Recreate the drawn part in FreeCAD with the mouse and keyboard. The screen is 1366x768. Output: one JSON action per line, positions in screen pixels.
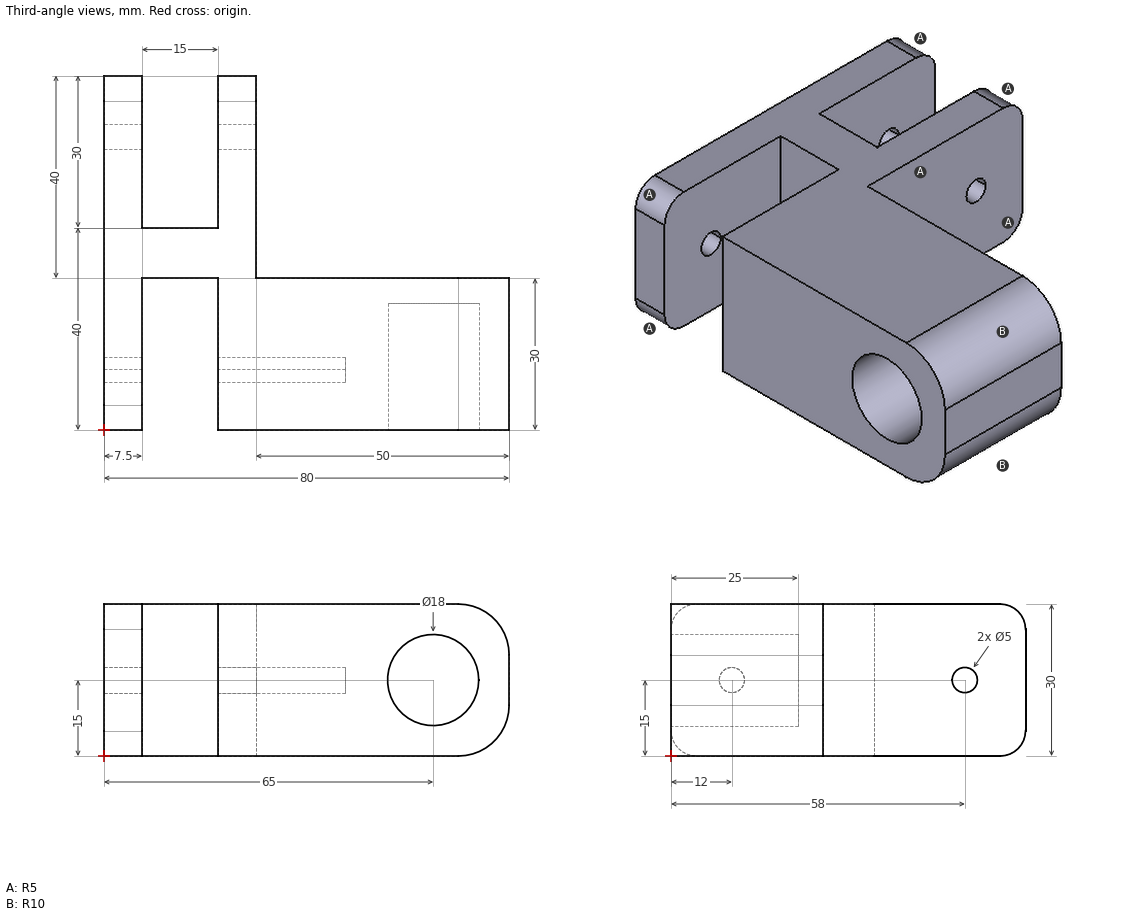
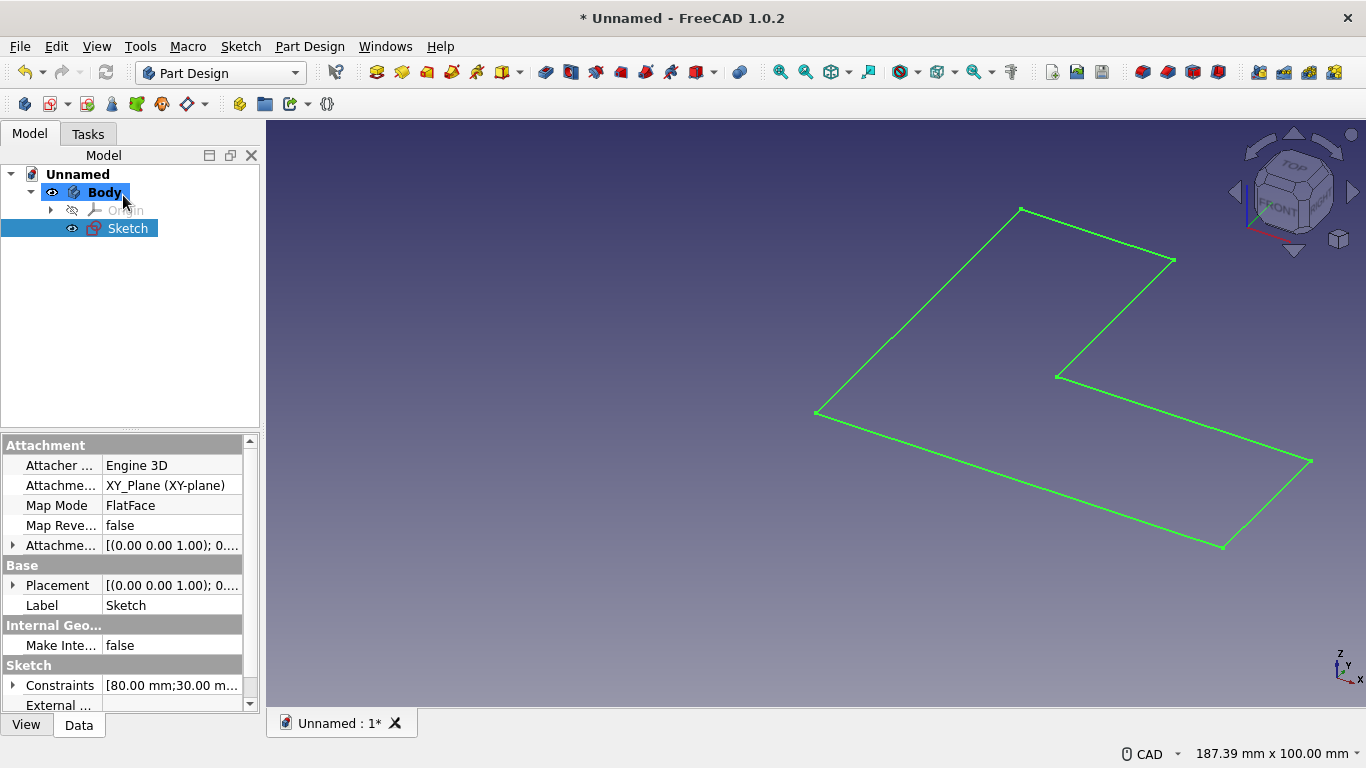
{"action": "left_click", "coordinate": [377, 72]}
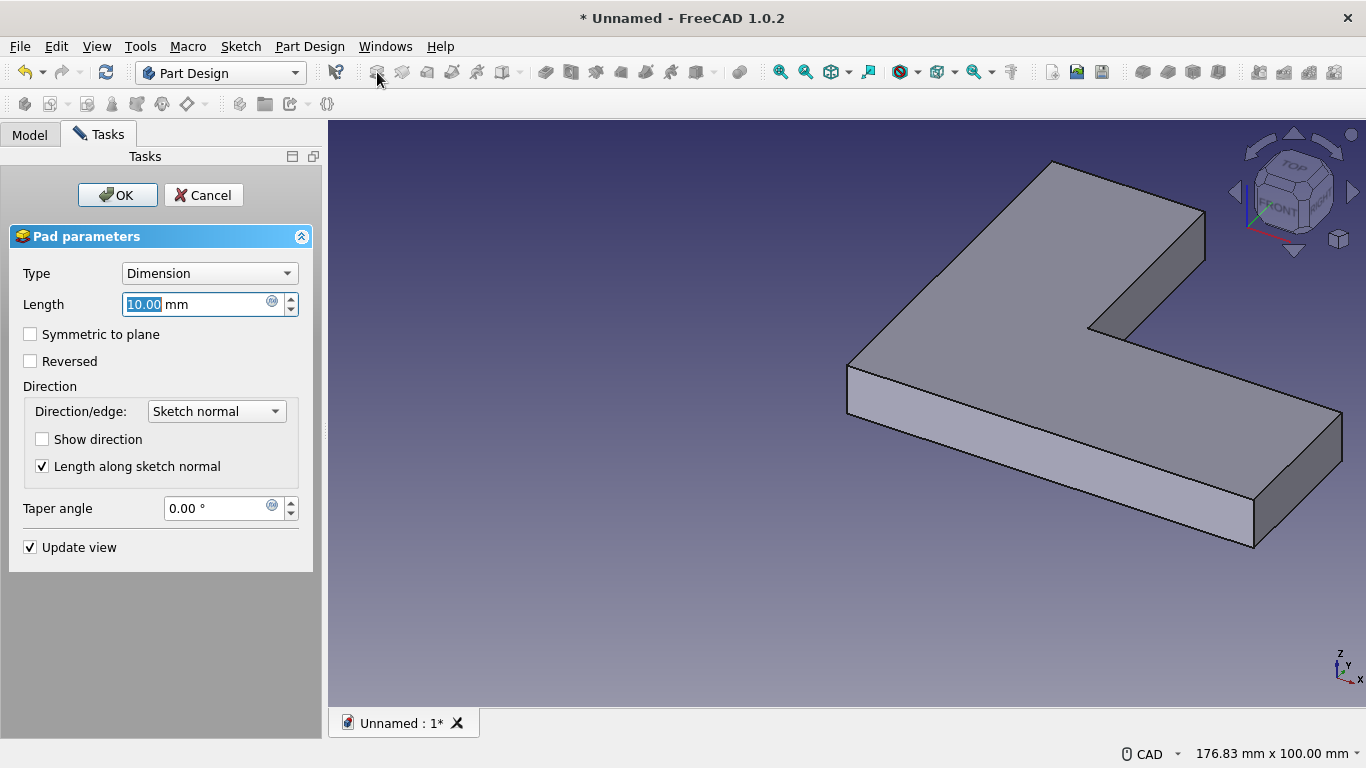
{"action": "type", "text": "30"}
{"action": "key", "text": "Tab"}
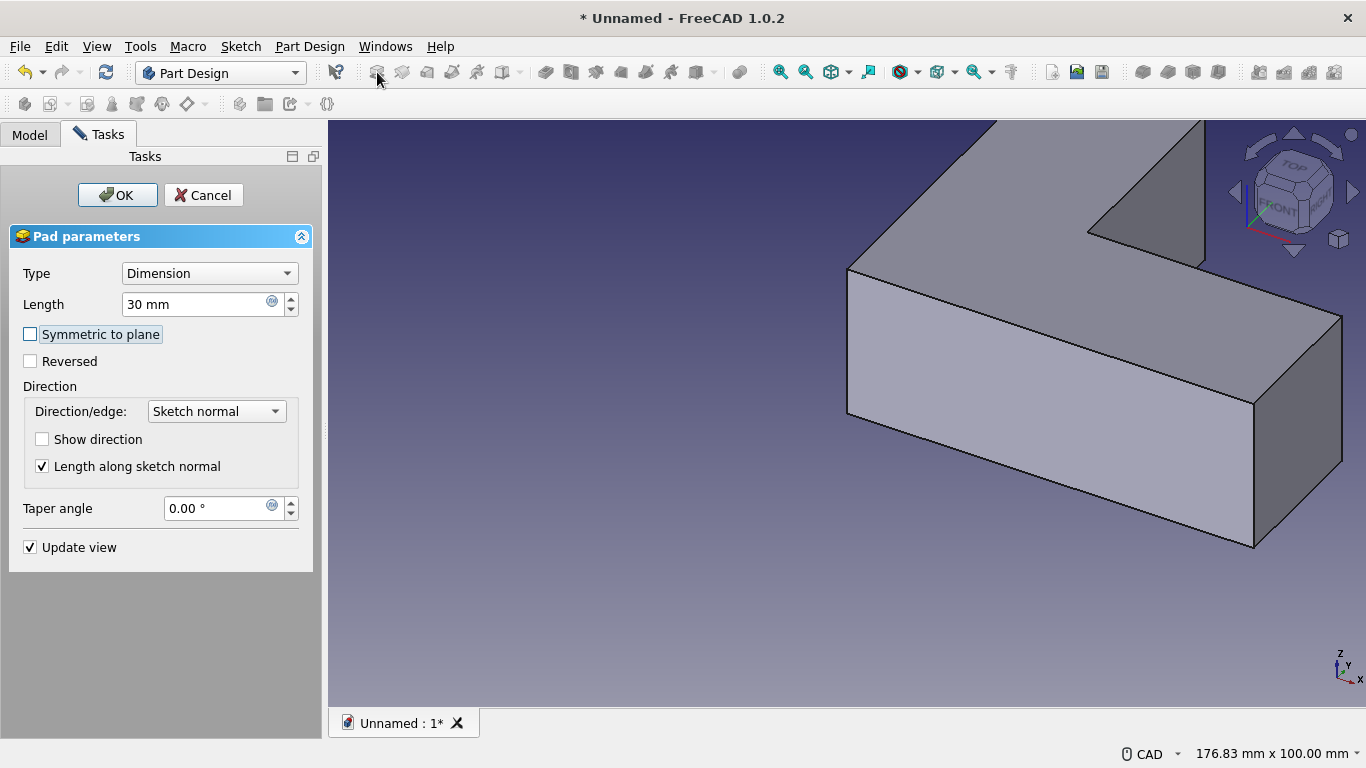
{"action": "left_click", "coordinate": [118, 195]}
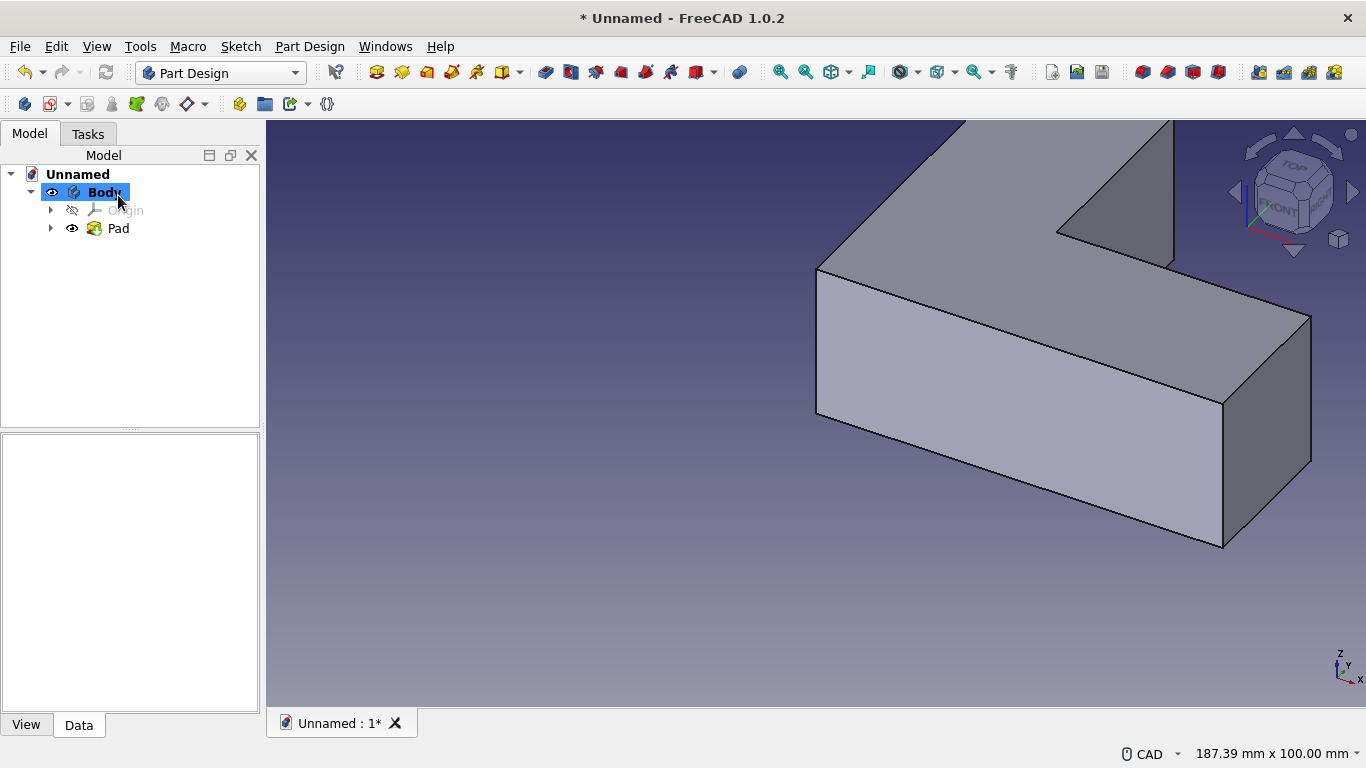
{"action": "left_click", "coordinate": [781, 72]}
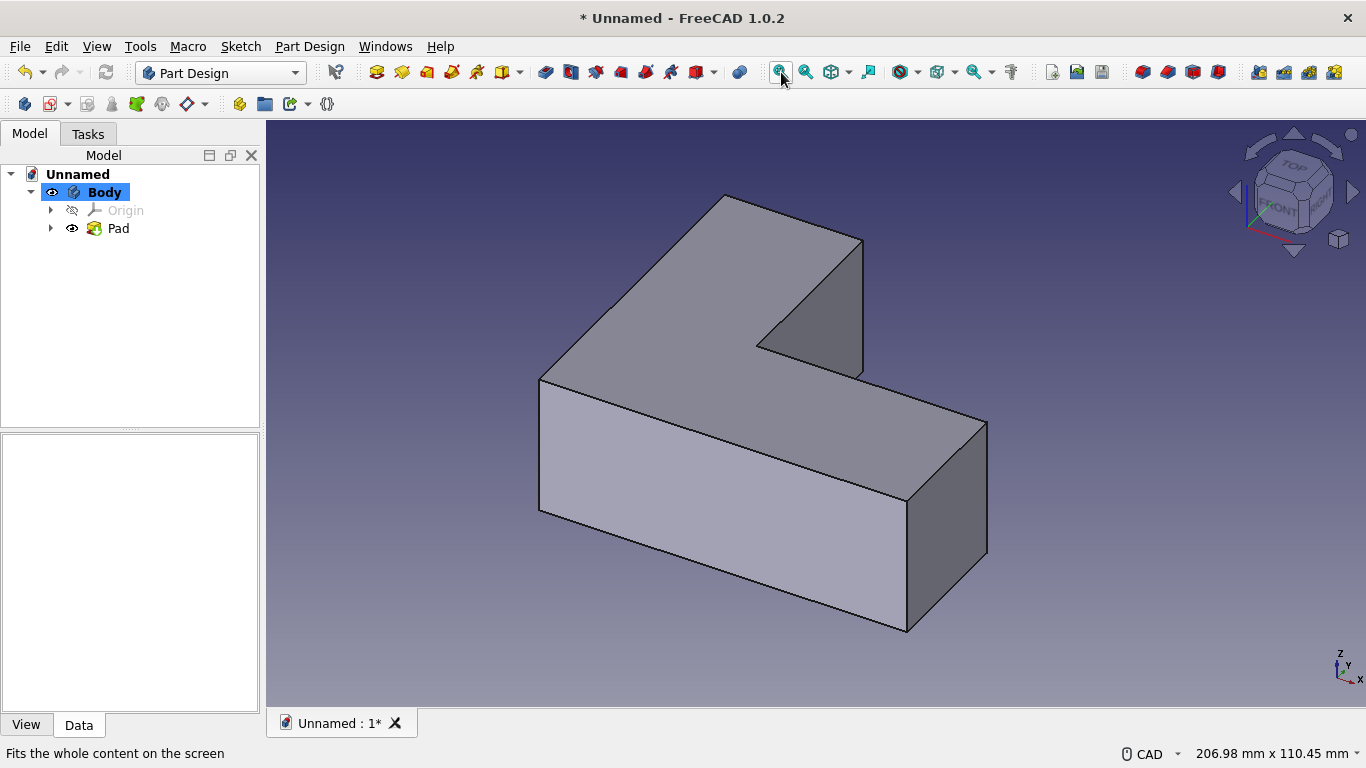
{"action": "left_click", "coordinate": [828, 540]}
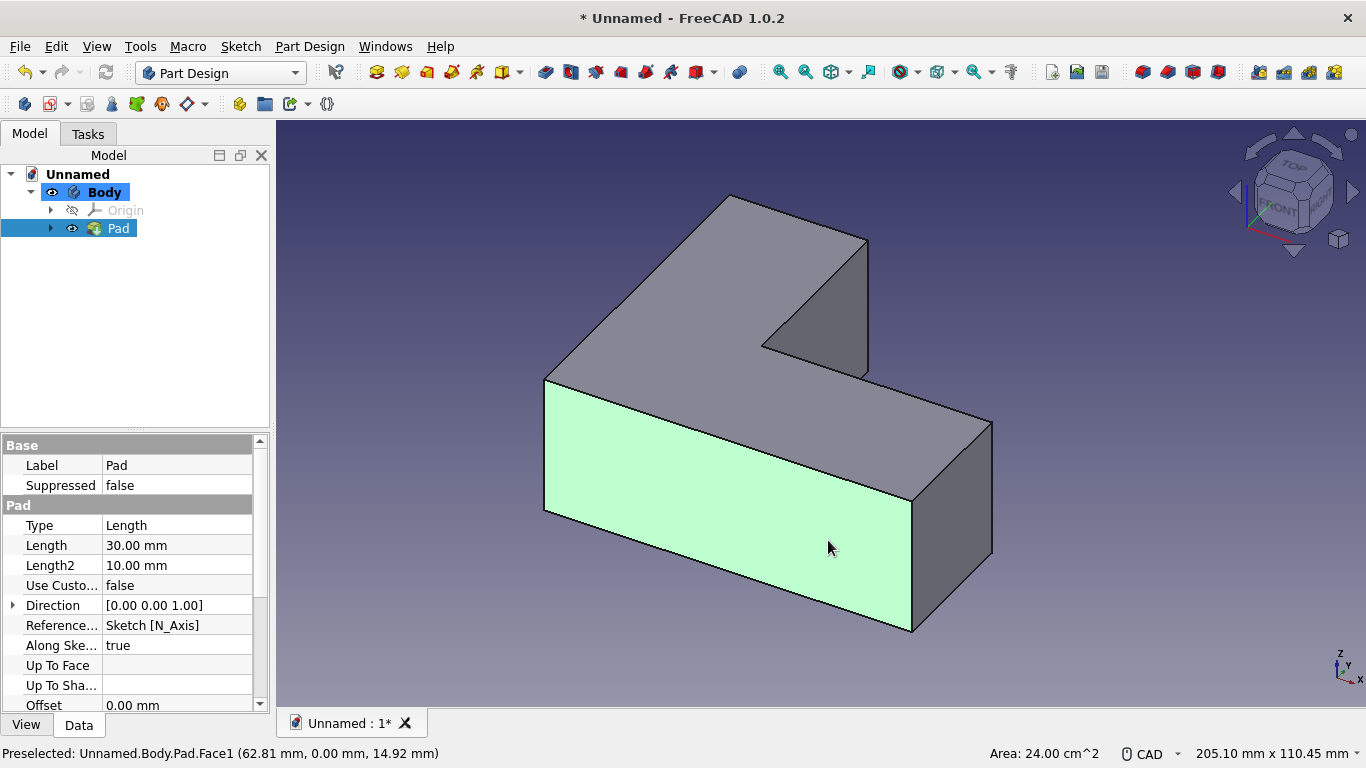
{"action": "left_click", "coordinate": [50, 104]}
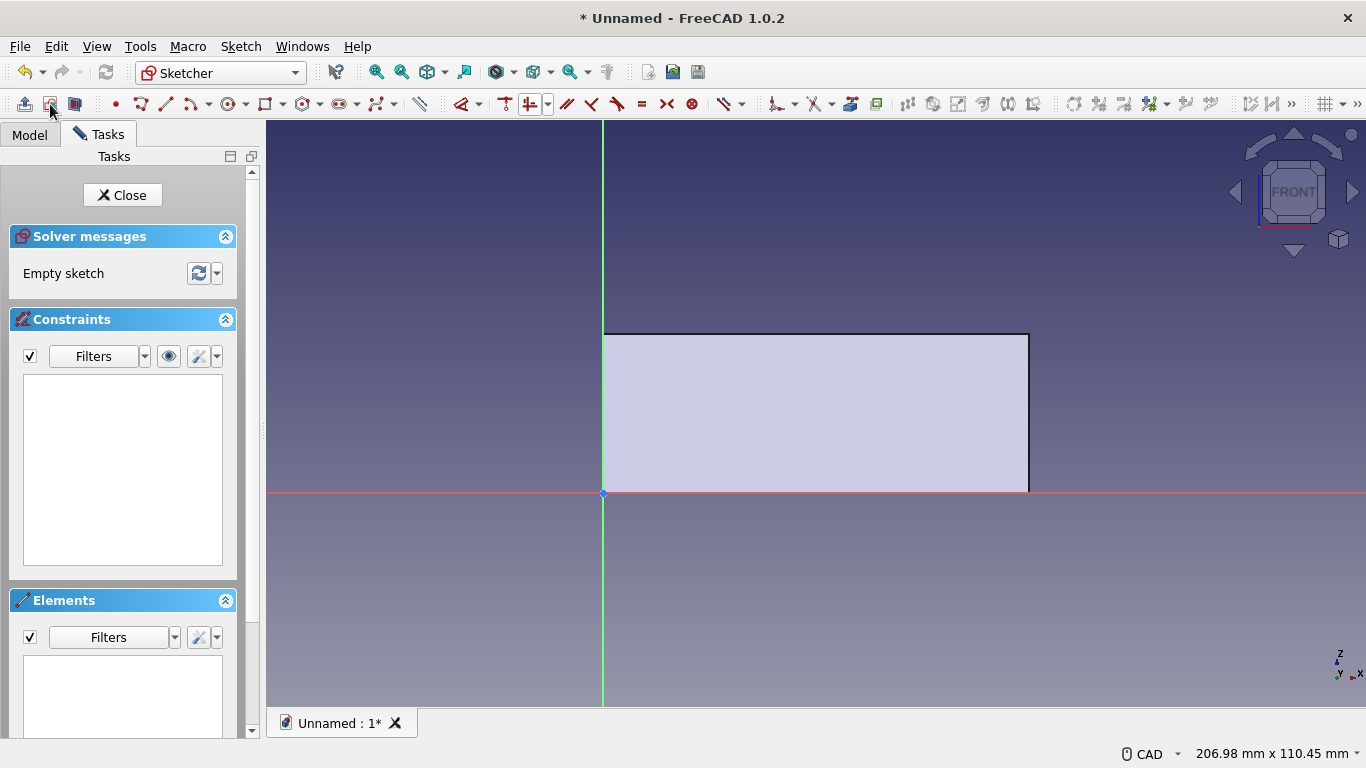
{"action": "scroll", "coordinate": [1015, 414], "scroll_direction": "up", "scroll_amount": 7}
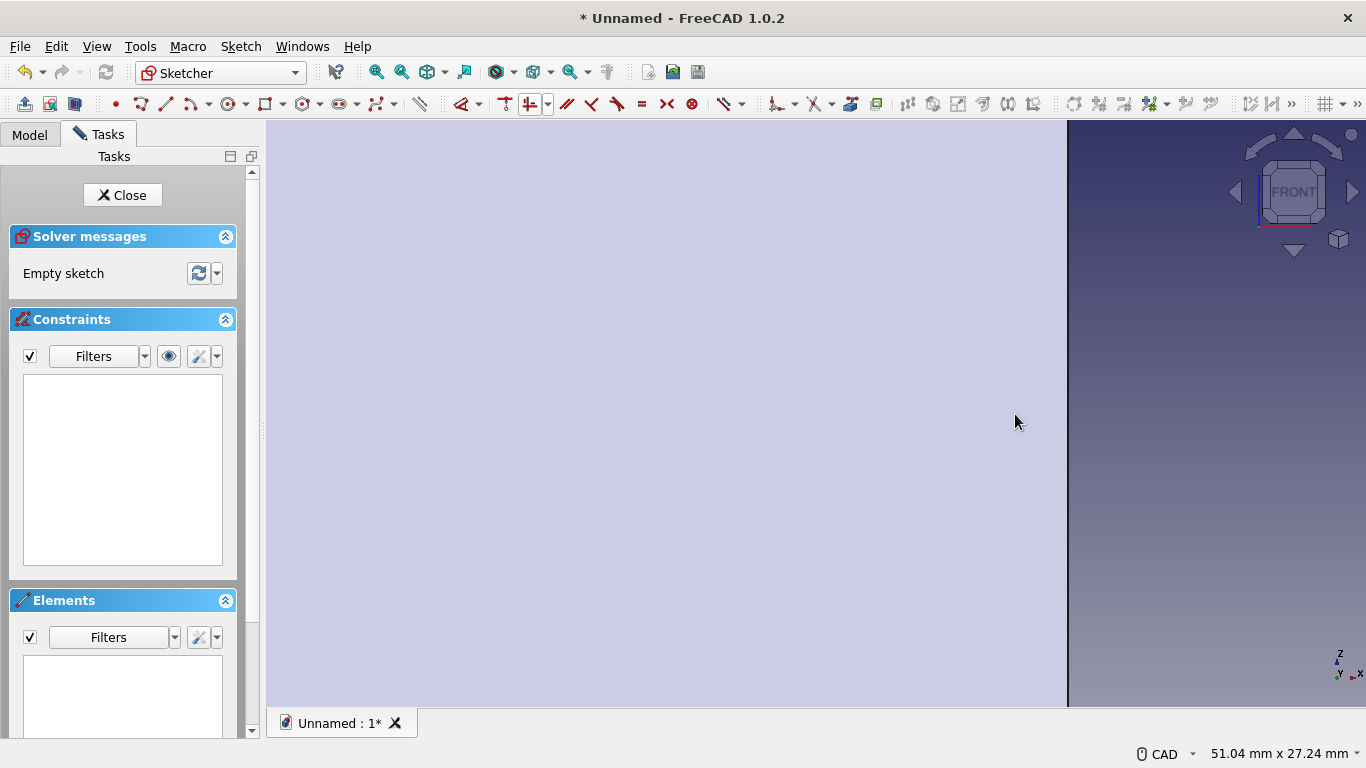
{"action": "key", "text": "g c"}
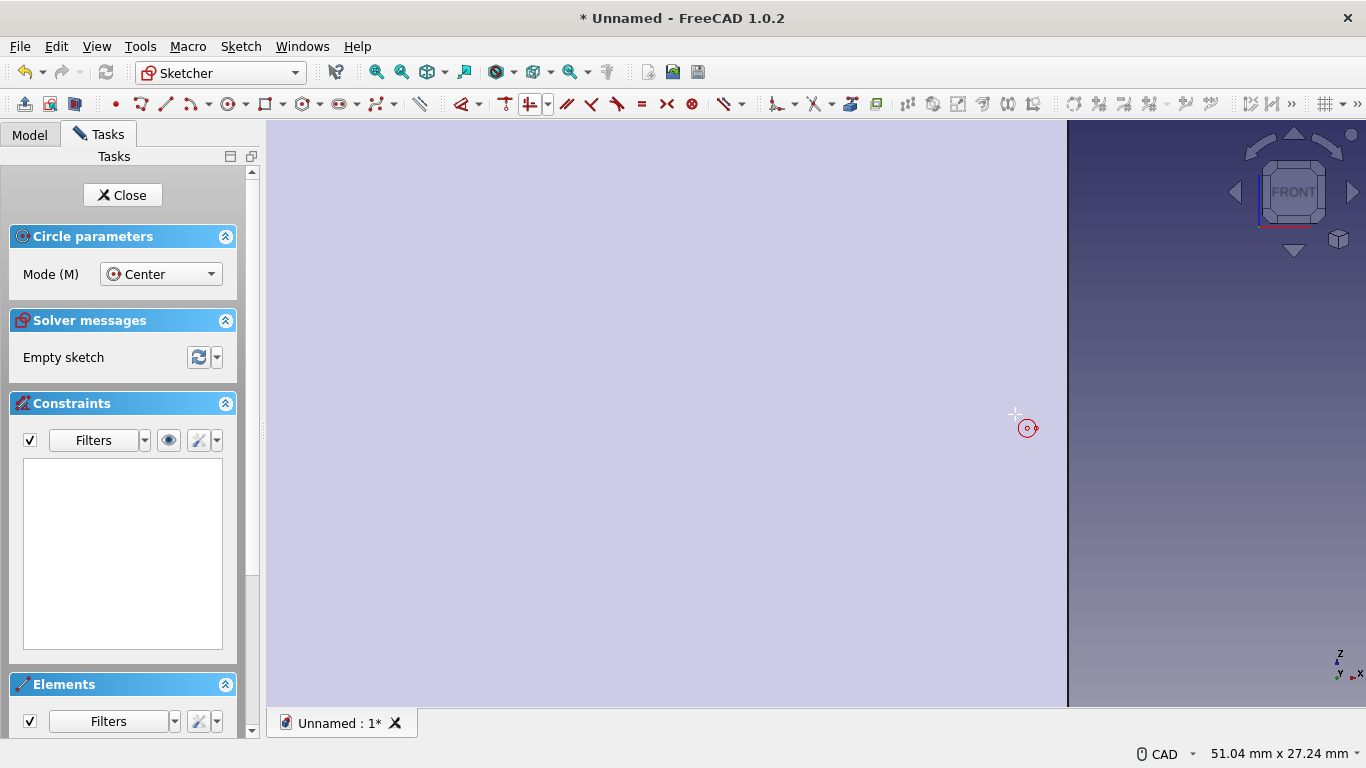
{"action": "left_click", "coordinate": [745, 410]}
{"action": "left_click", "coordinate": [882, 273]}
{"action": "key", "text": "Escape"}